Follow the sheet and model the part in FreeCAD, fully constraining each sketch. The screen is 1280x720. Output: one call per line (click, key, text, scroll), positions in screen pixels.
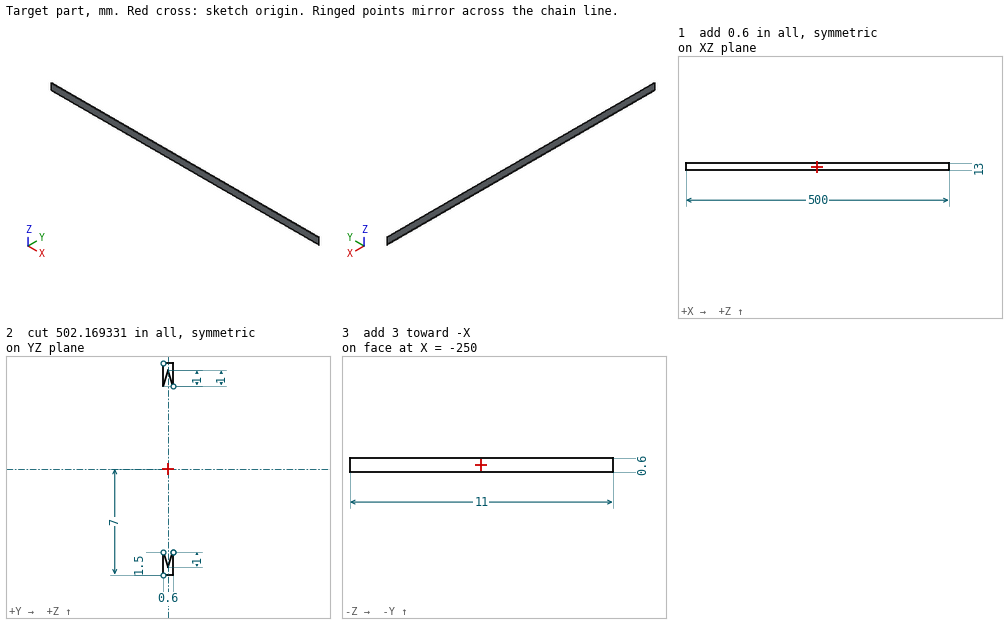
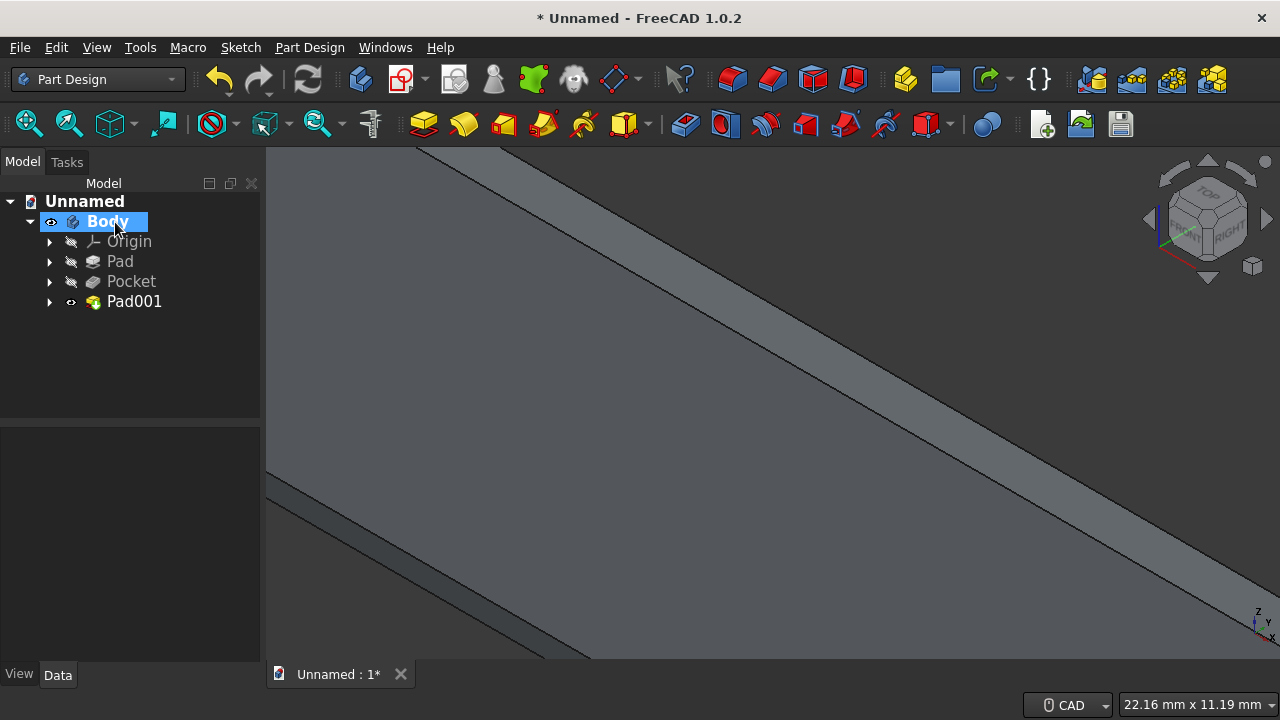
key(v)
key(f)